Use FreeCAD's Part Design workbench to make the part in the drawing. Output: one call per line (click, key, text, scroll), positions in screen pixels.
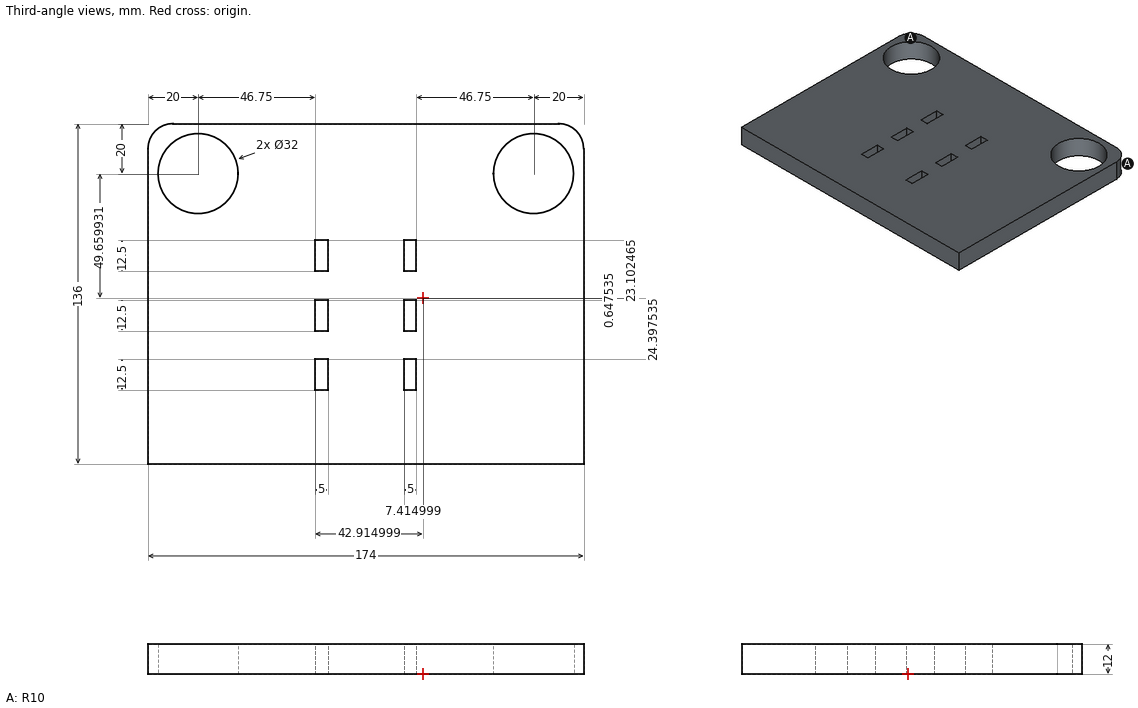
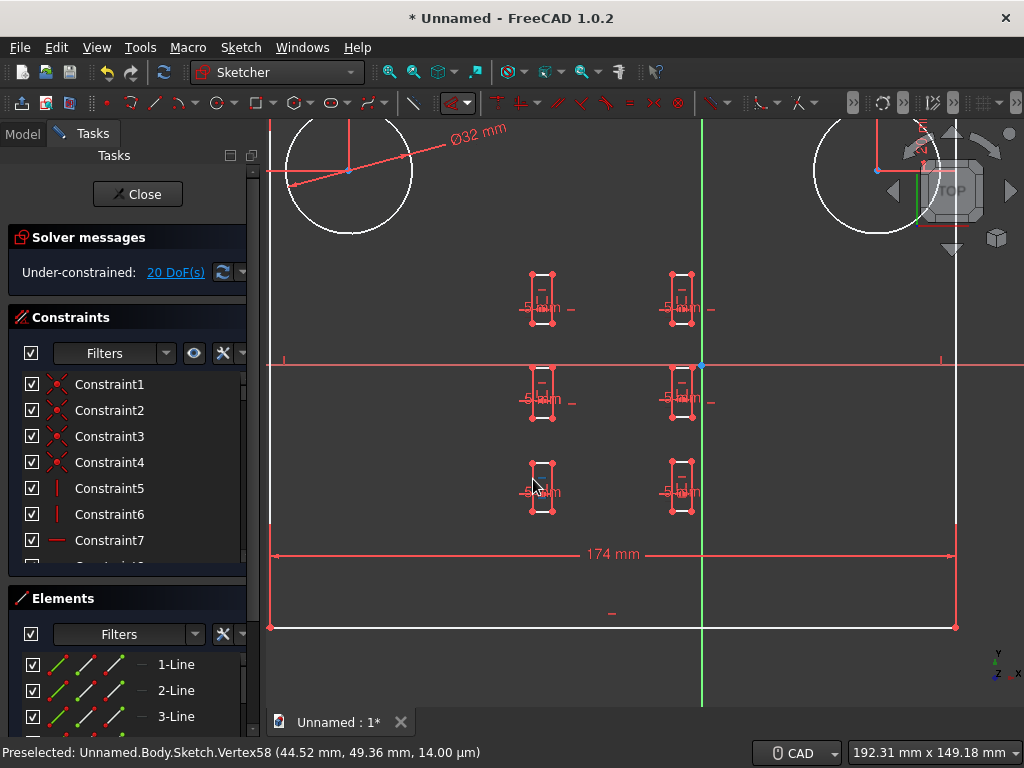
click(533, 478)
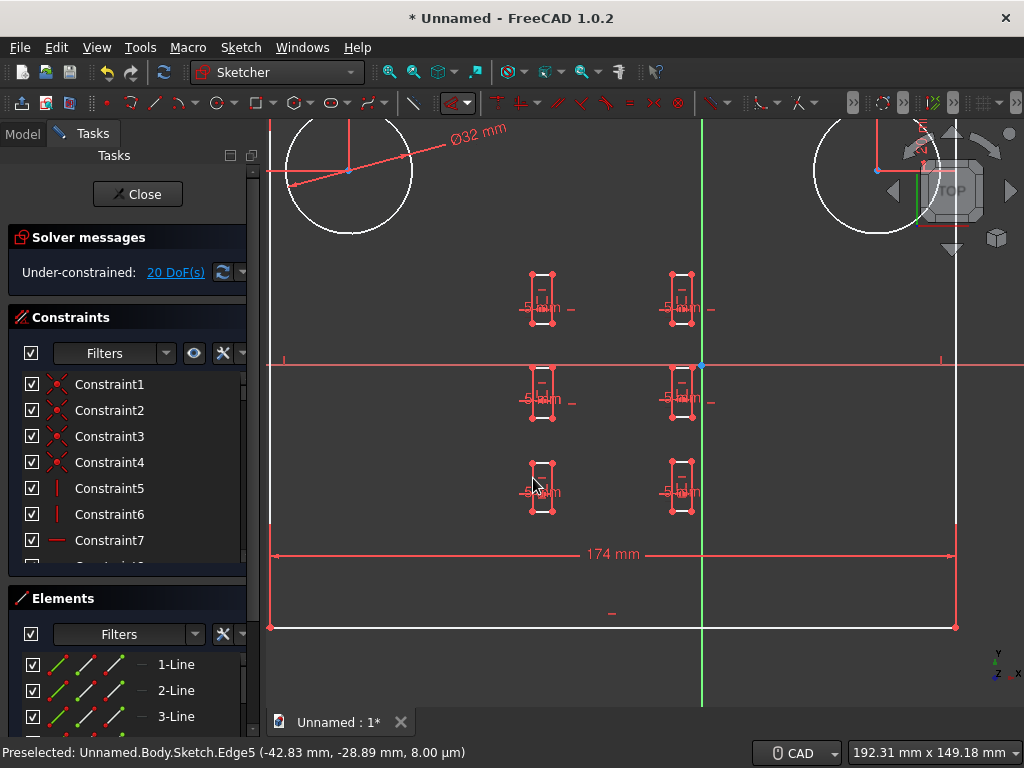
click(470, 104)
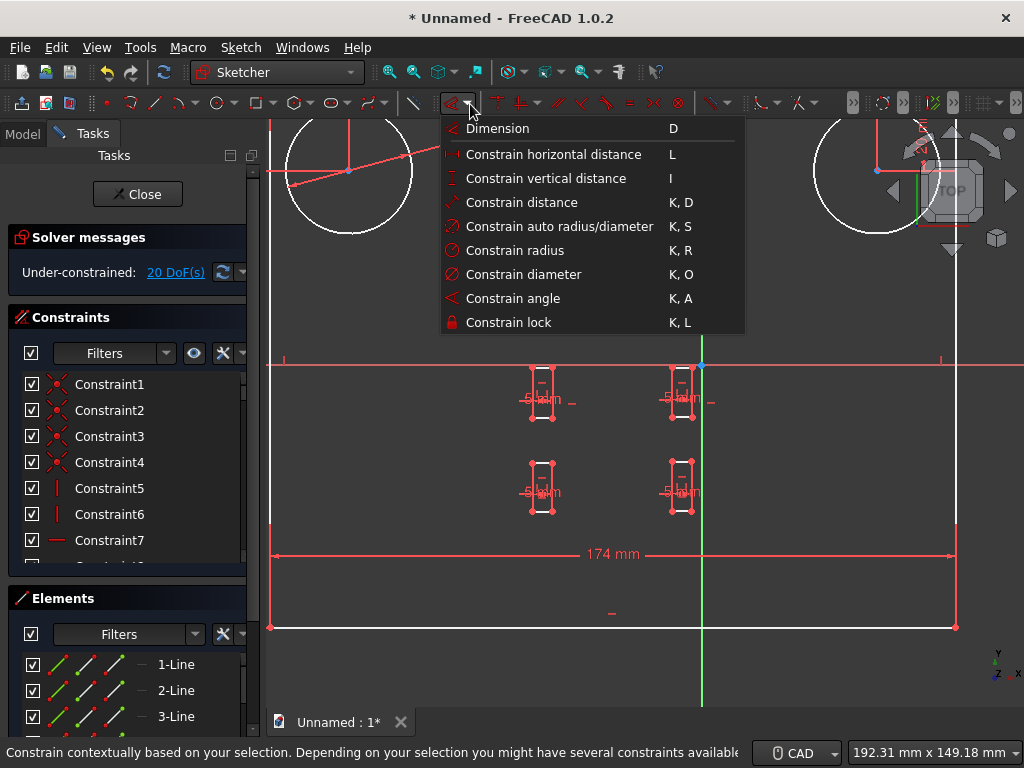
click(593, 178)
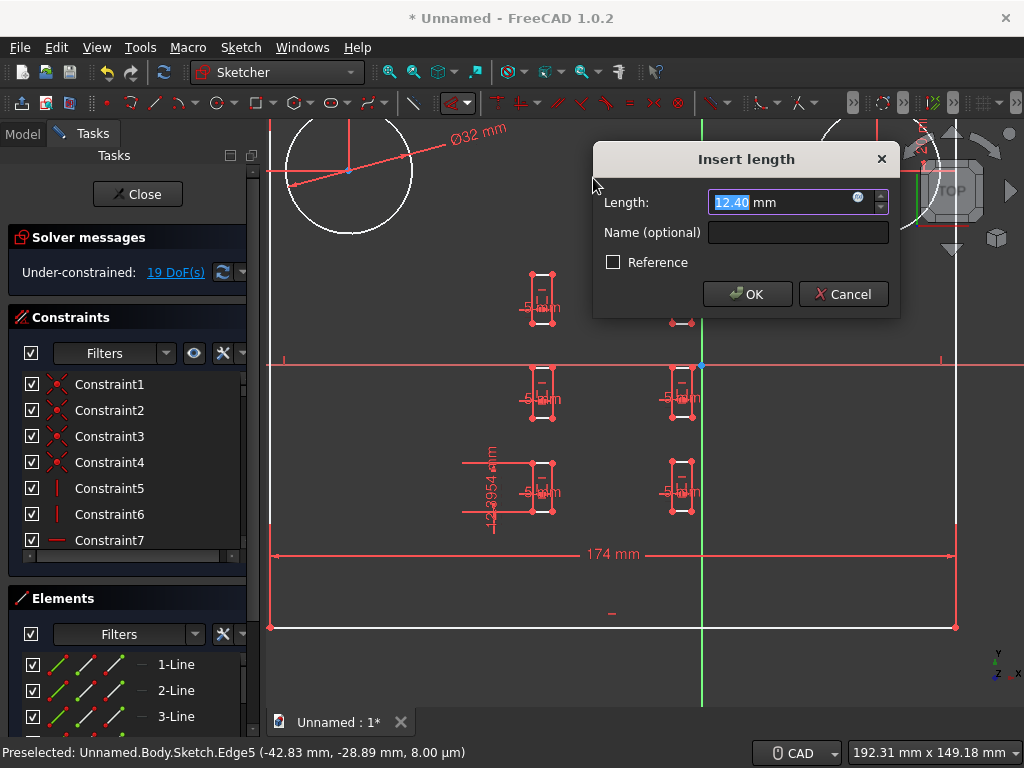
text(12.5)
key(Return)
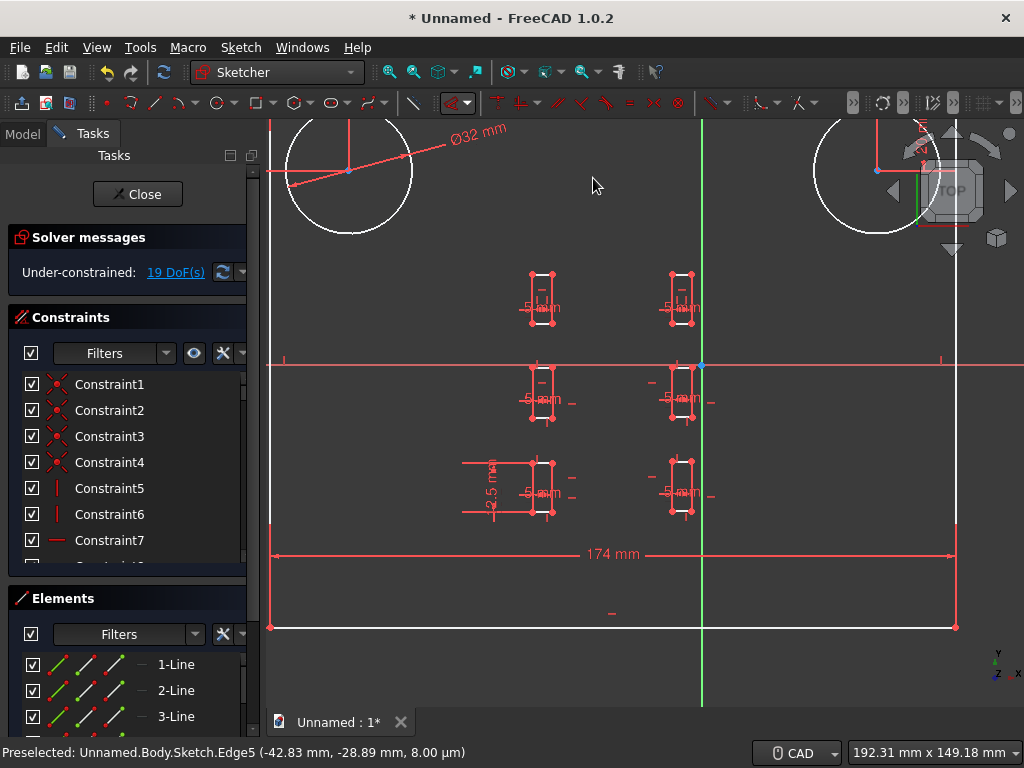
click(533, 383)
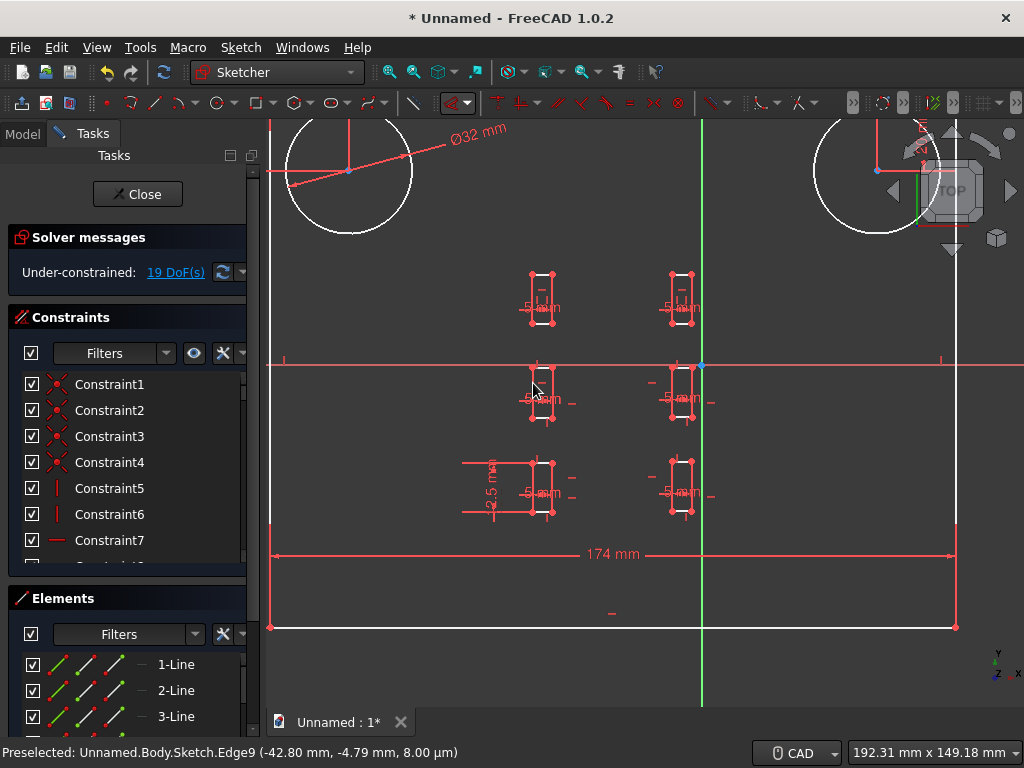
key(i)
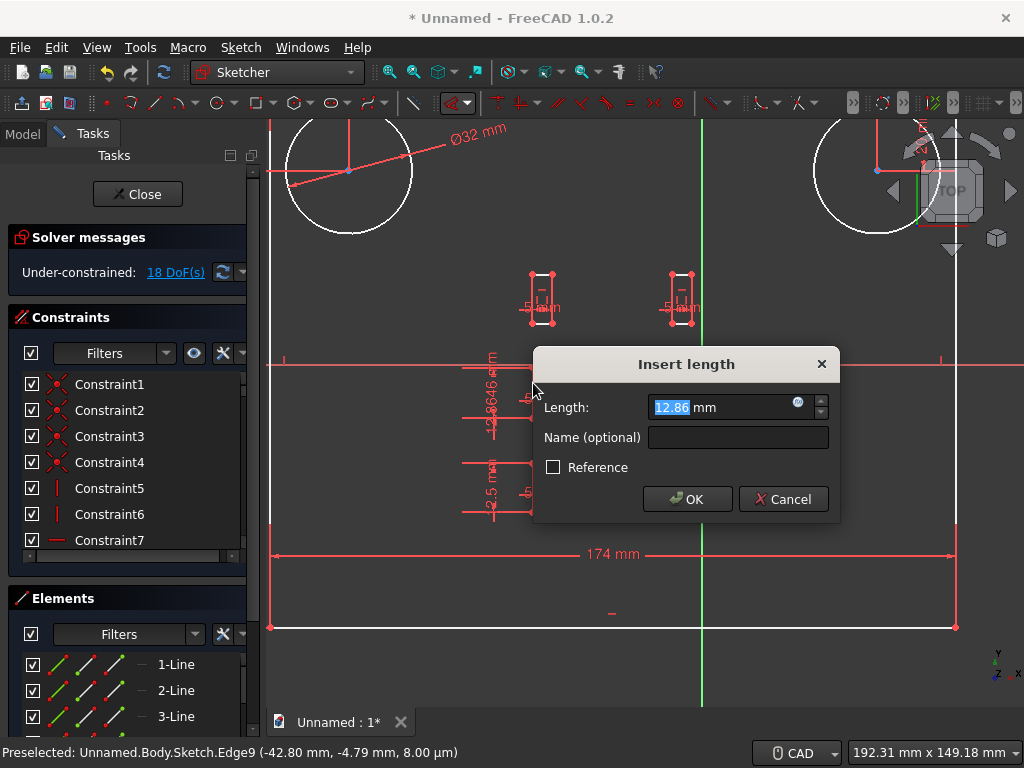
text(12.5)
key(Return)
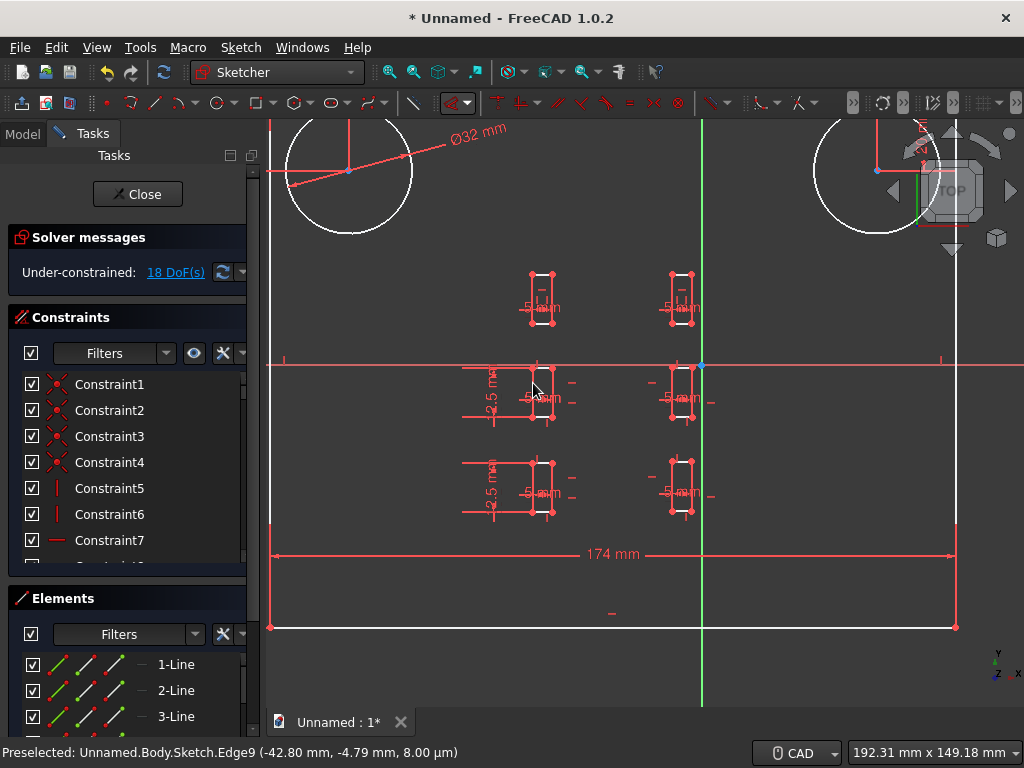
click(672, 477)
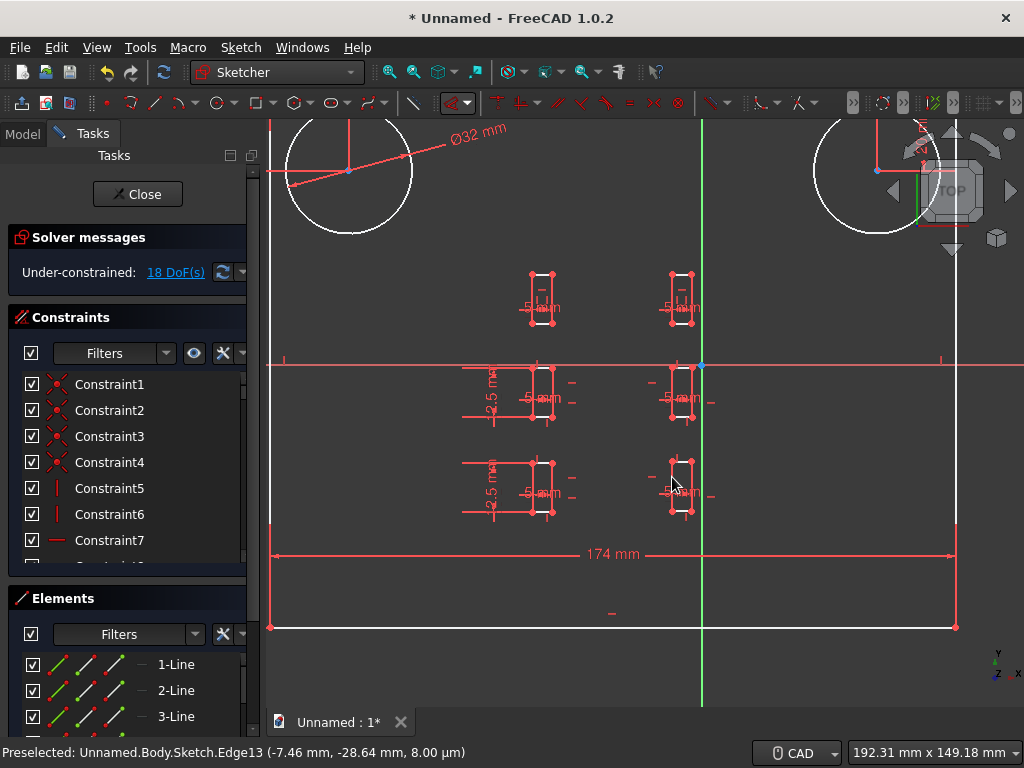
click(470, 104)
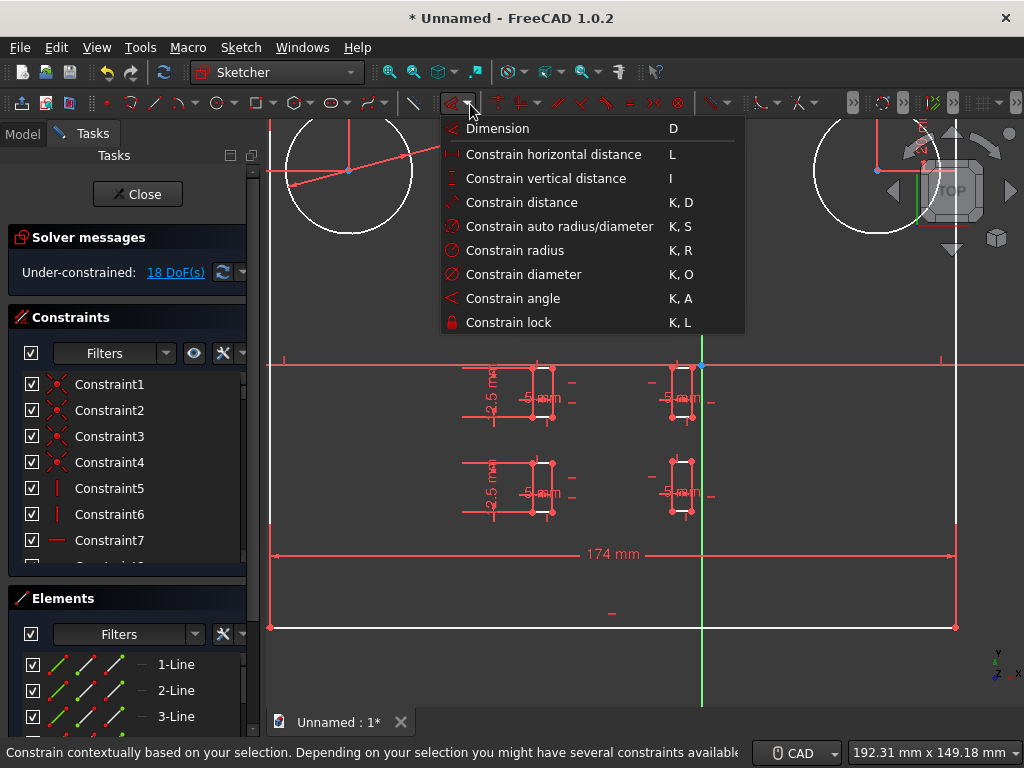
click(593, 178)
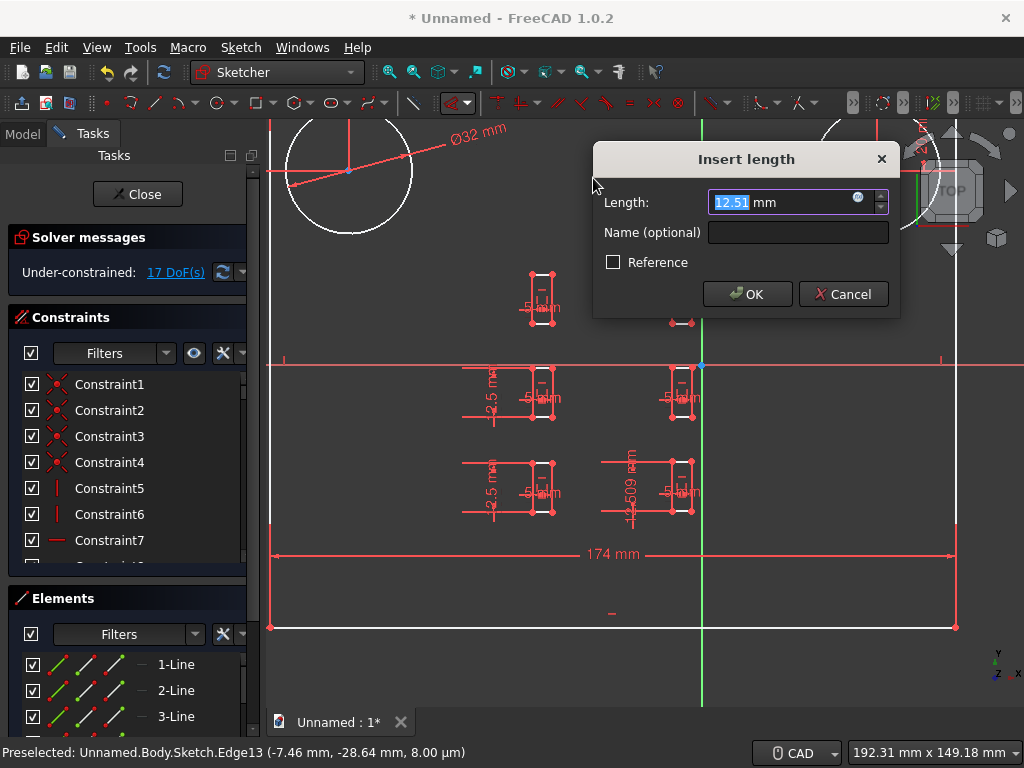
text(12.5)
key(Return)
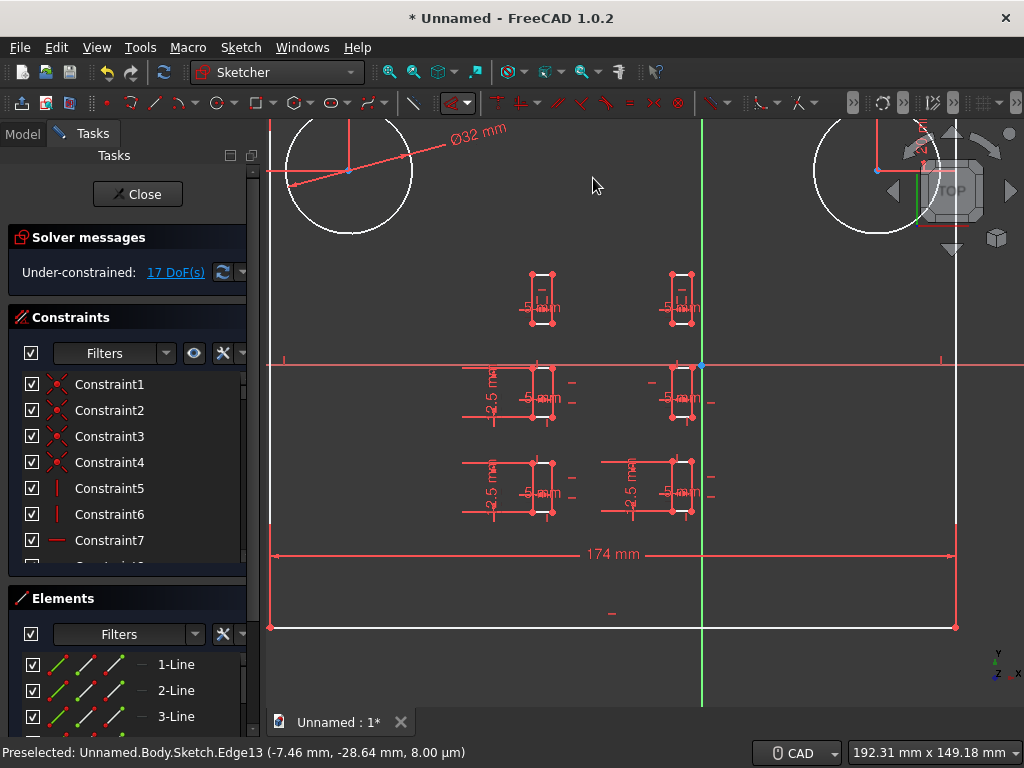
click(672, 383)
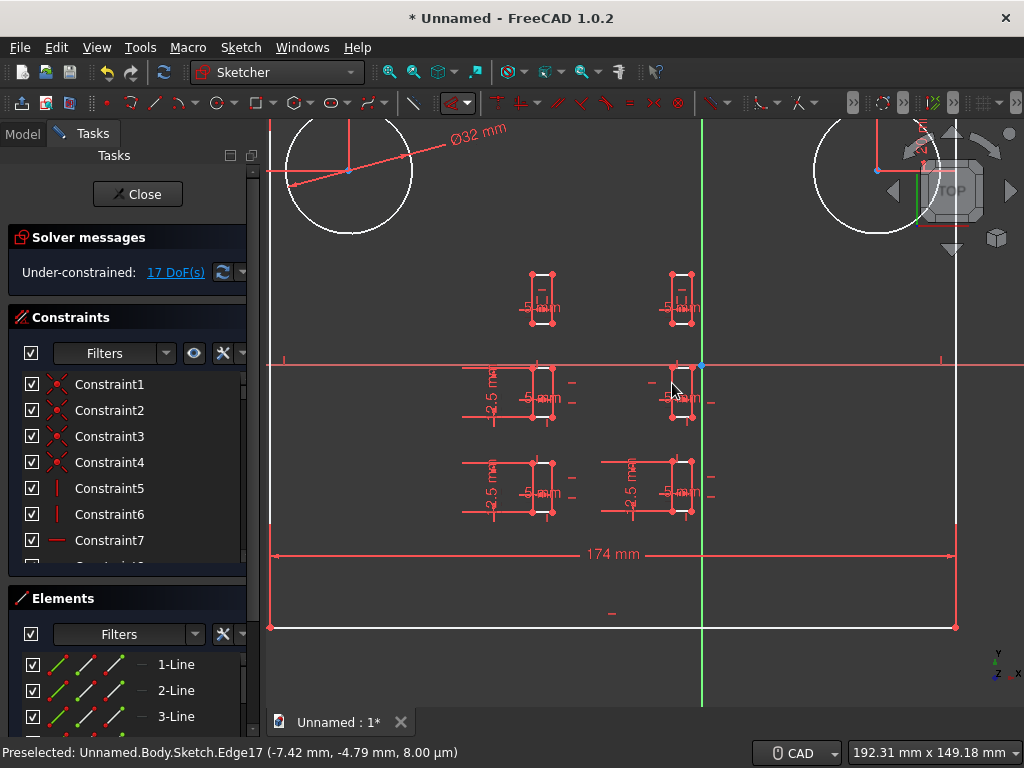
key(i)